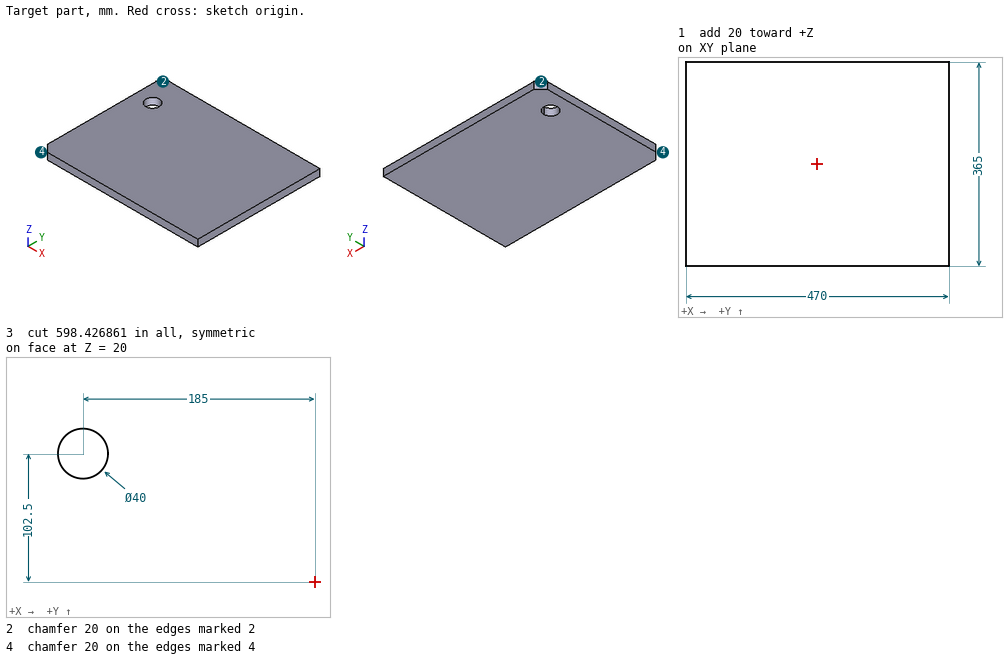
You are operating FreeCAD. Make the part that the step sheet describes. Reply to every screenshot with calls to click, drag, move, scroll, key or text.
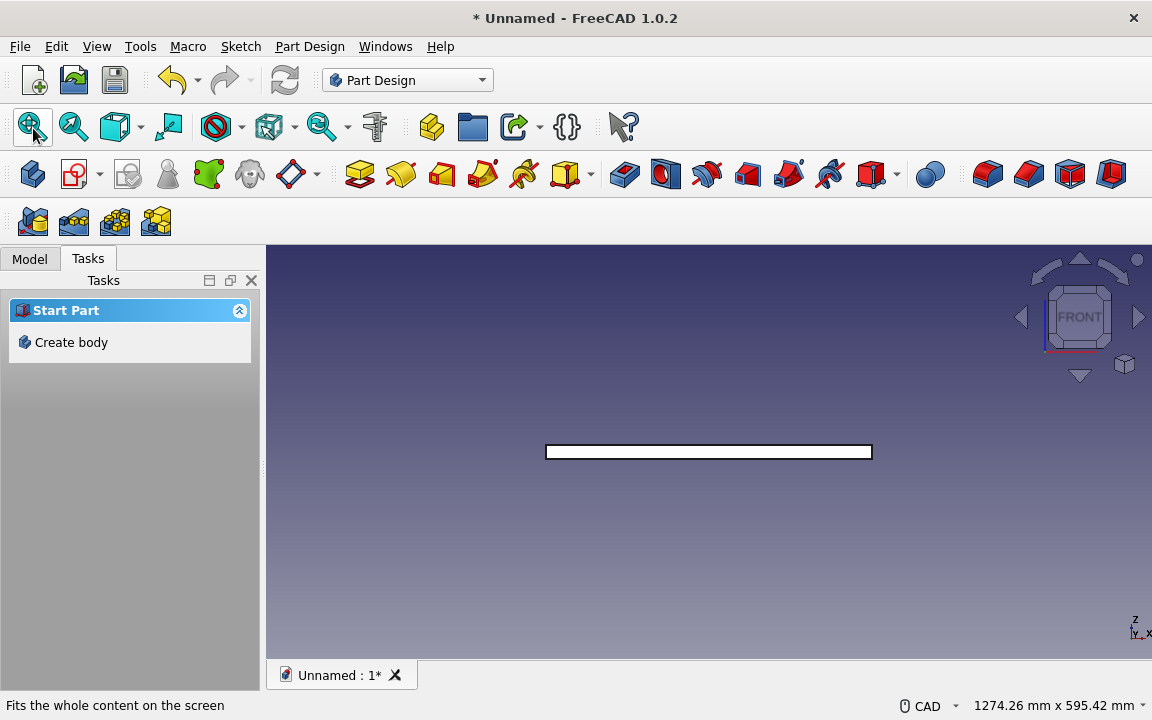
click(546, 451)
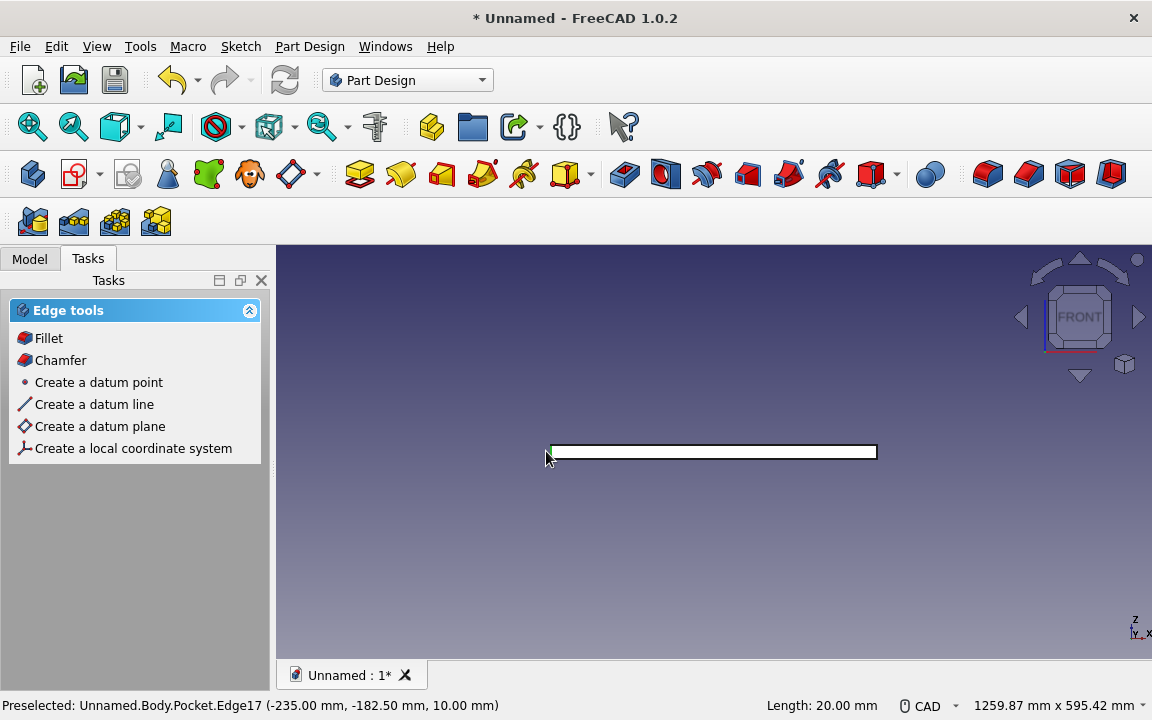
click(1029, 174)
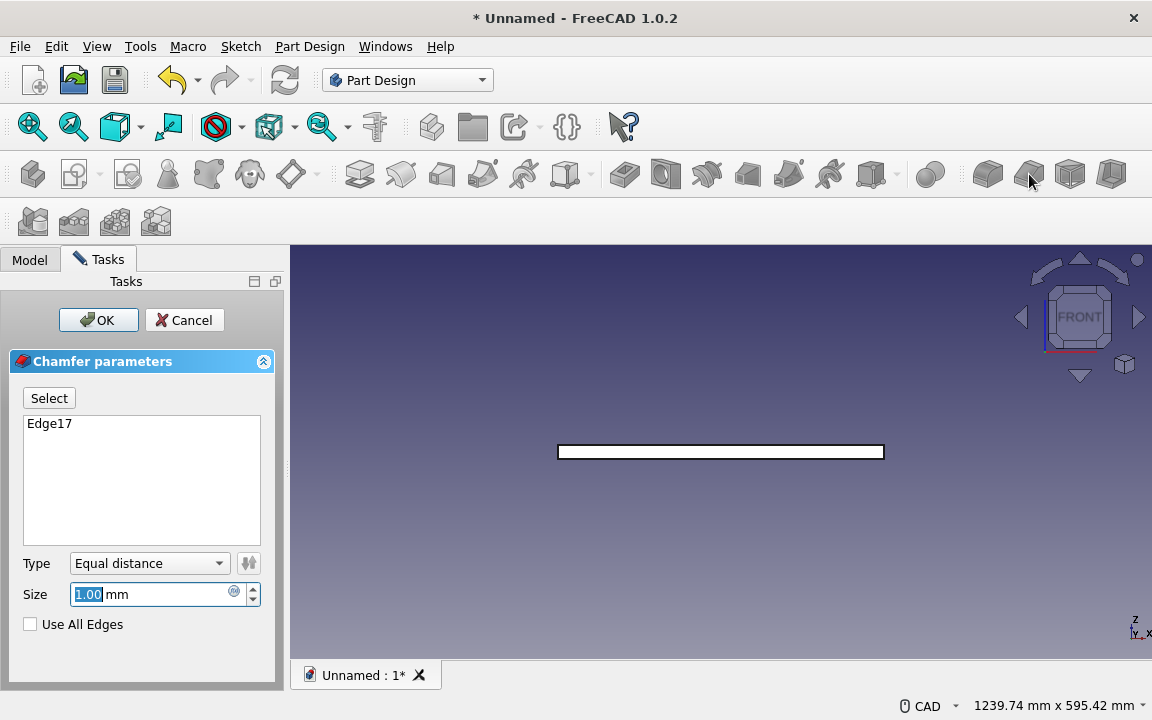
text(20)
key(Tab)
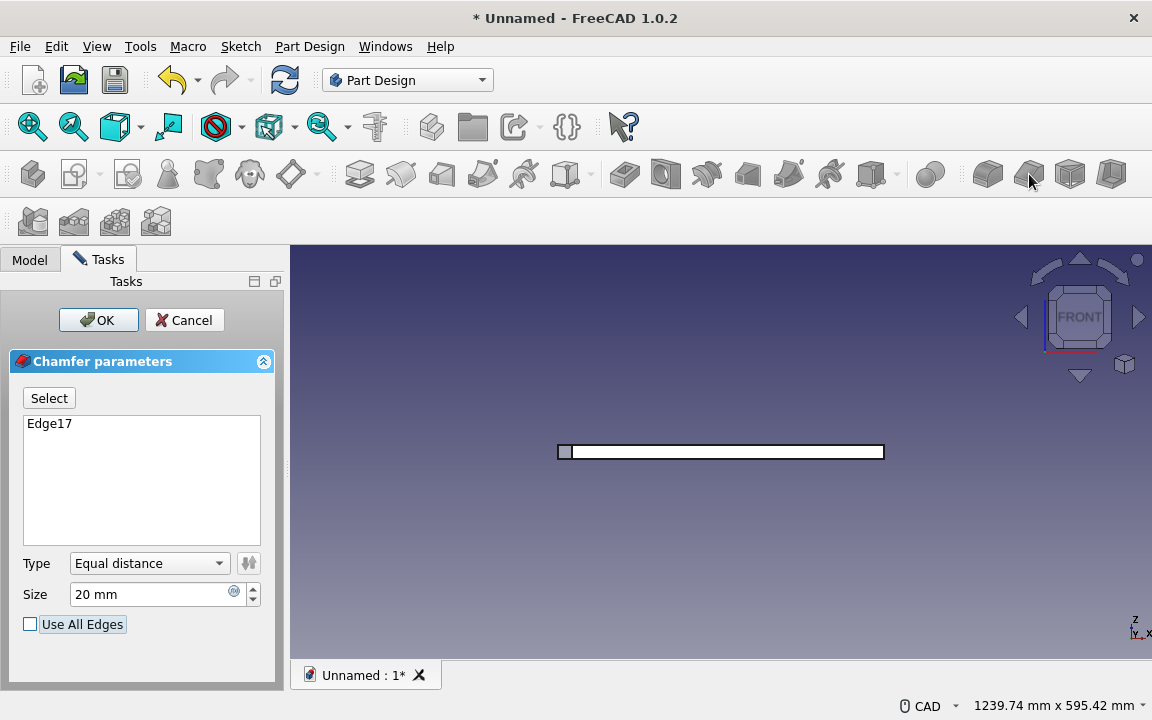
click(99, 320)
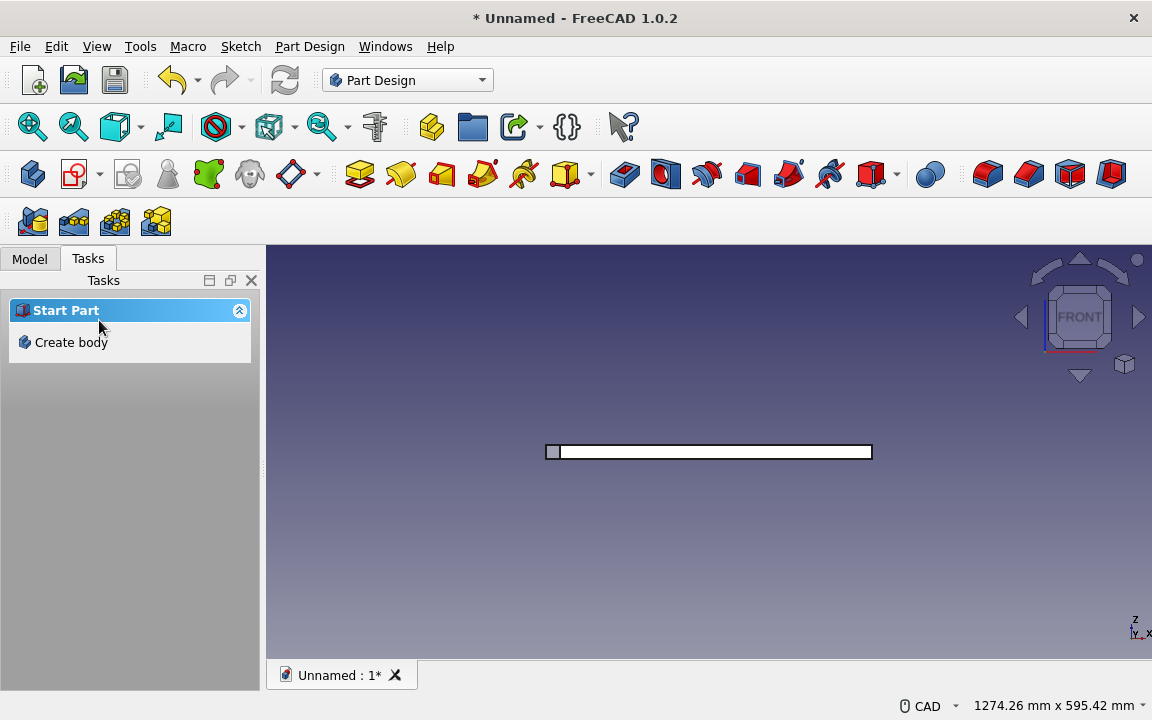
key(0)